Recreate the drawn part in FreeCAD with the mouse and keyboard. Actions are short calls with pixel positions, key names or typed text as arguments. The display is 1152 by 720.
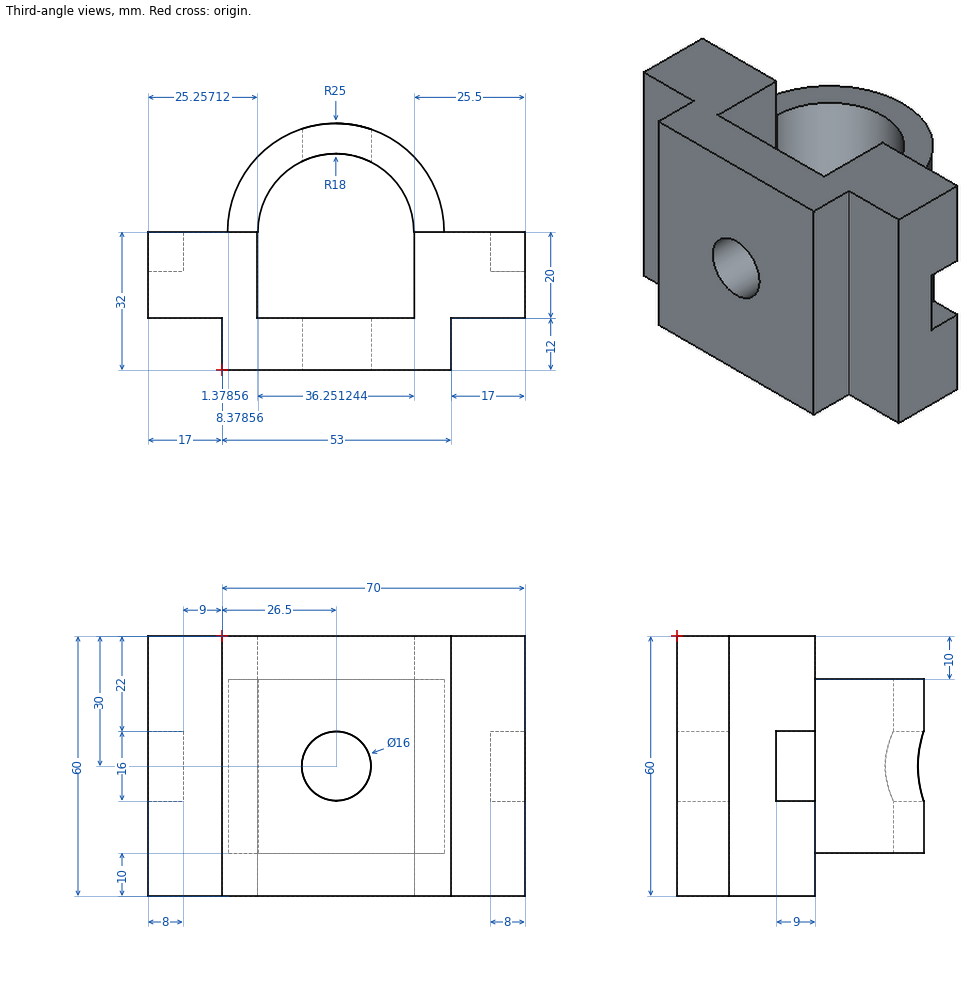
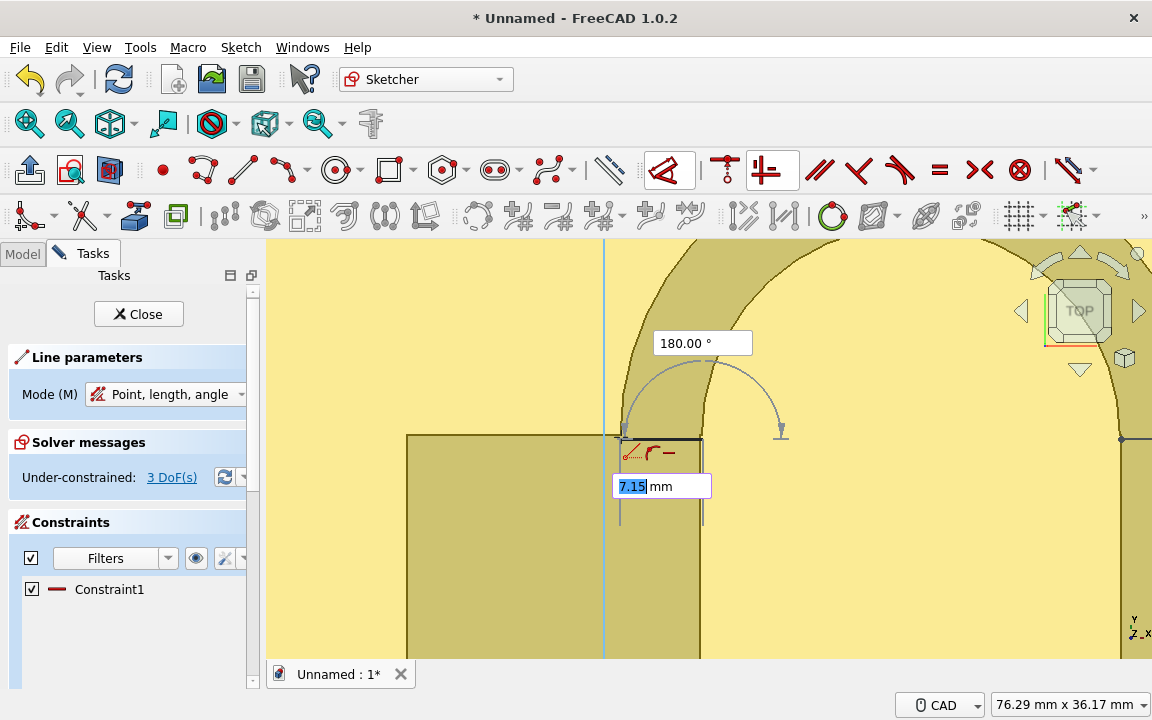
click(621, 436)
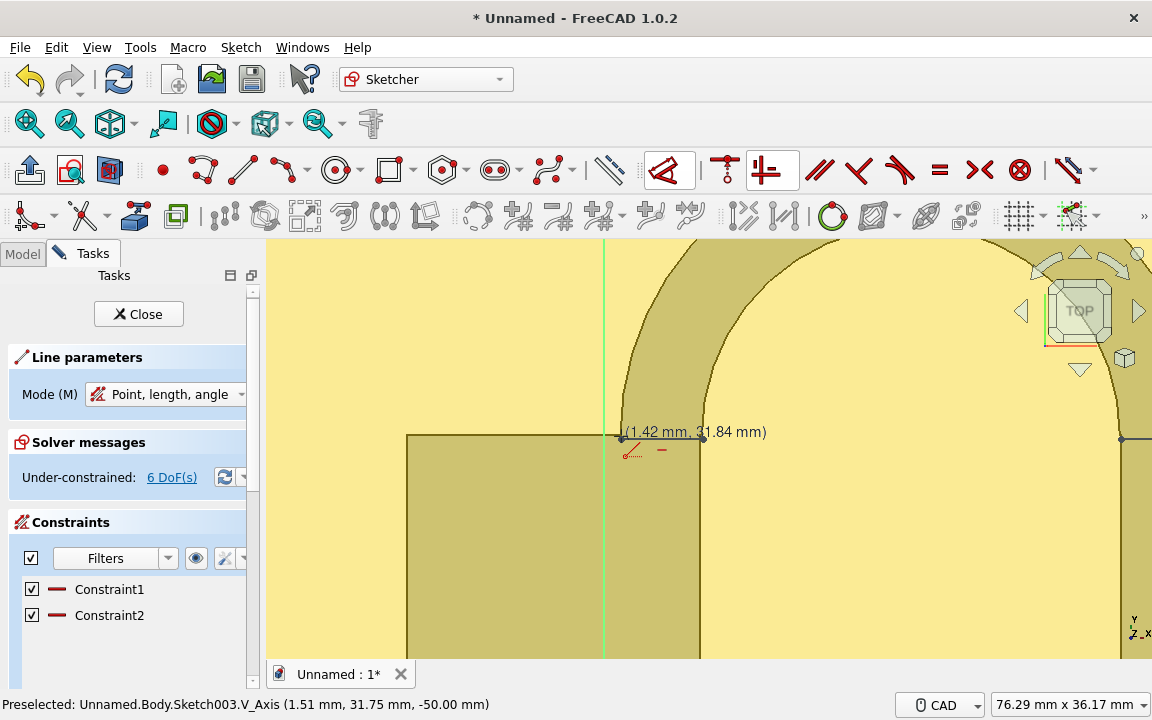
click(284, 170)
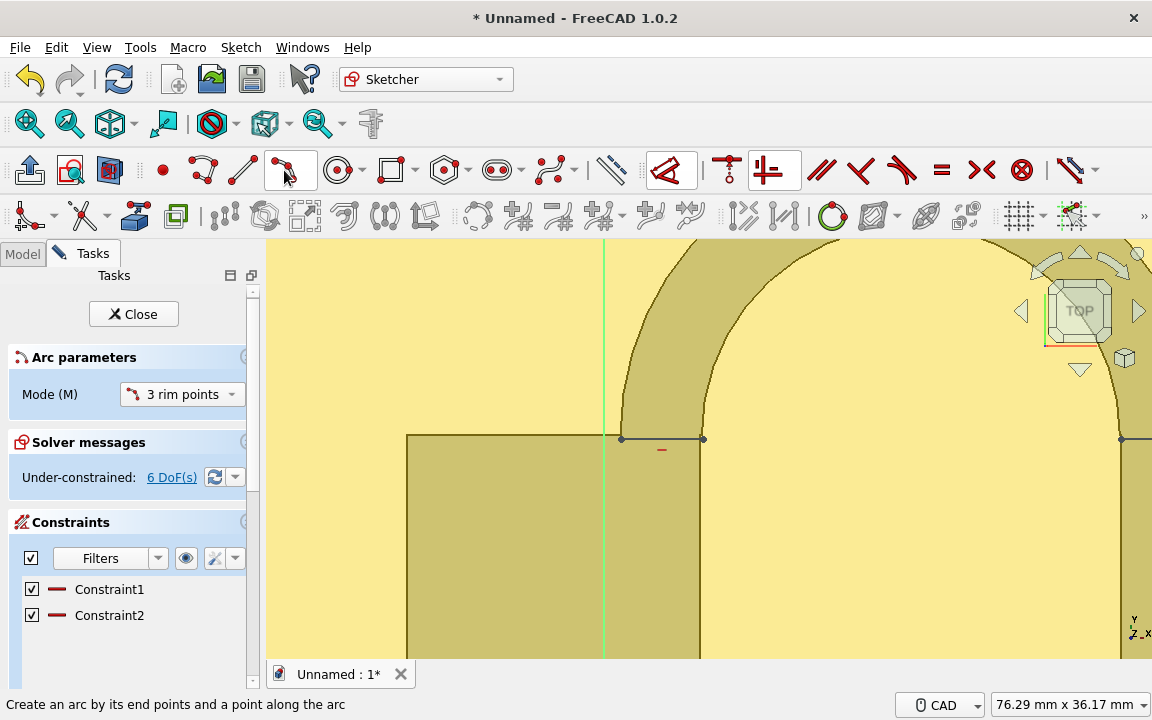
scroll(488, 433, down, 5)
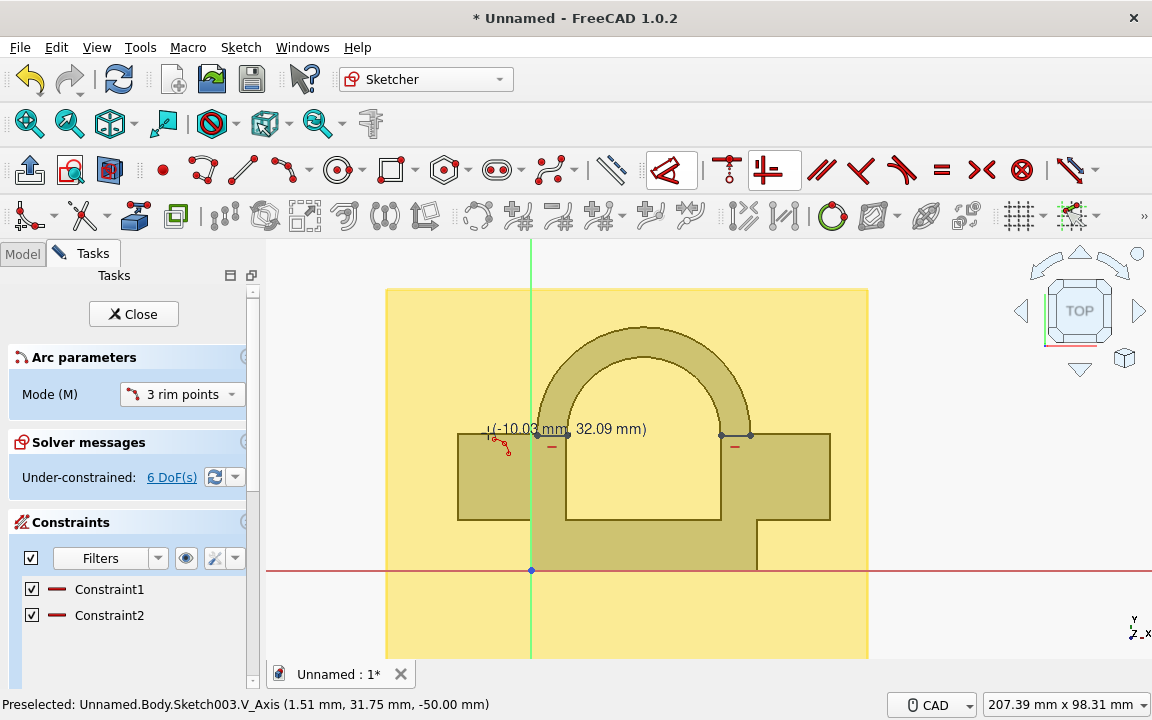
click(721, 436)
click(567, 436)
click(644, 357)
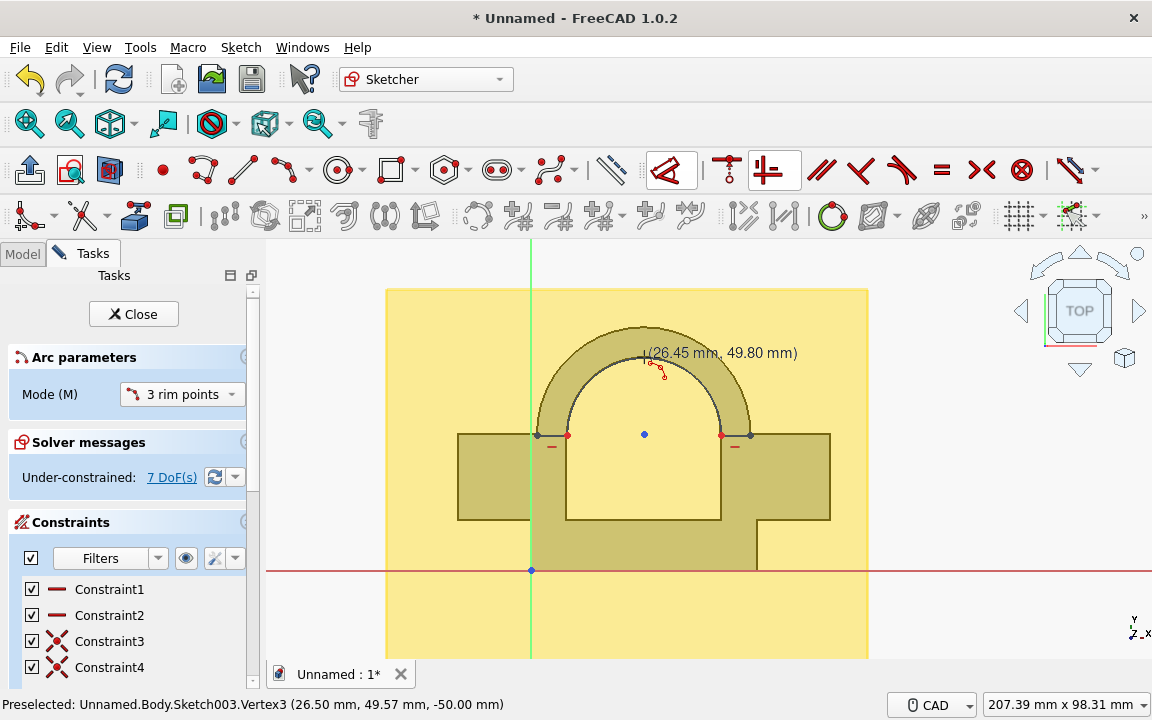
scroll(537, 434, up, 5)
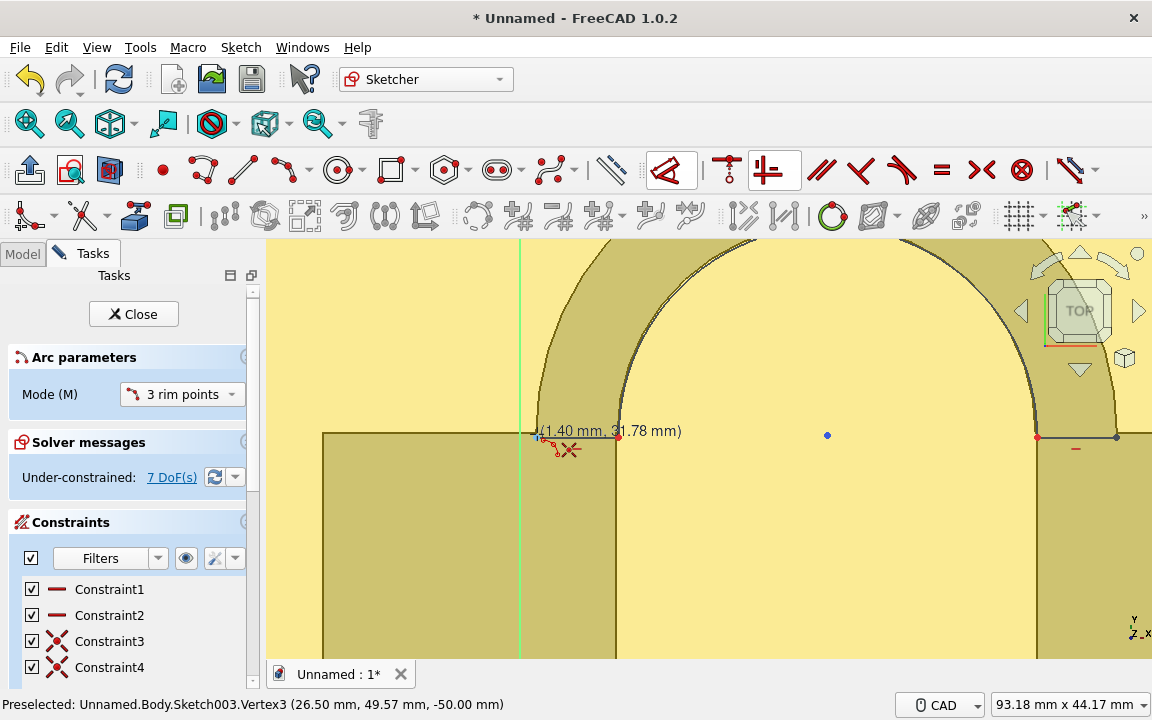
click(537, 438)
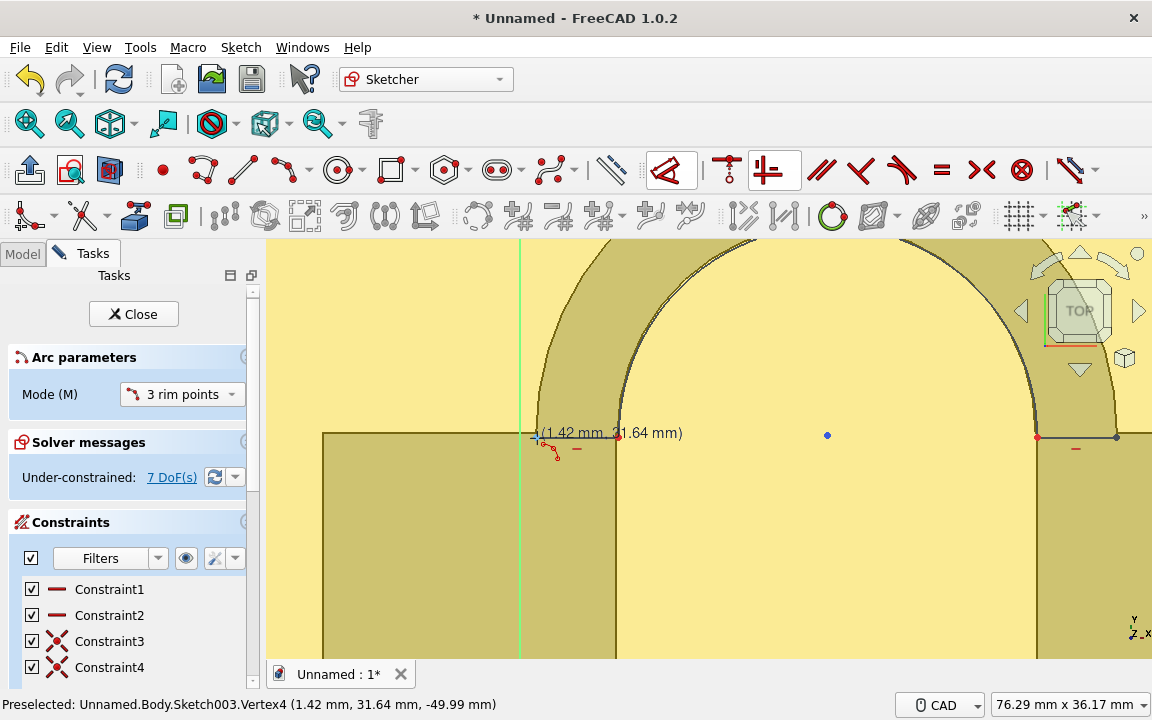
scroll(537, 434, down, 5)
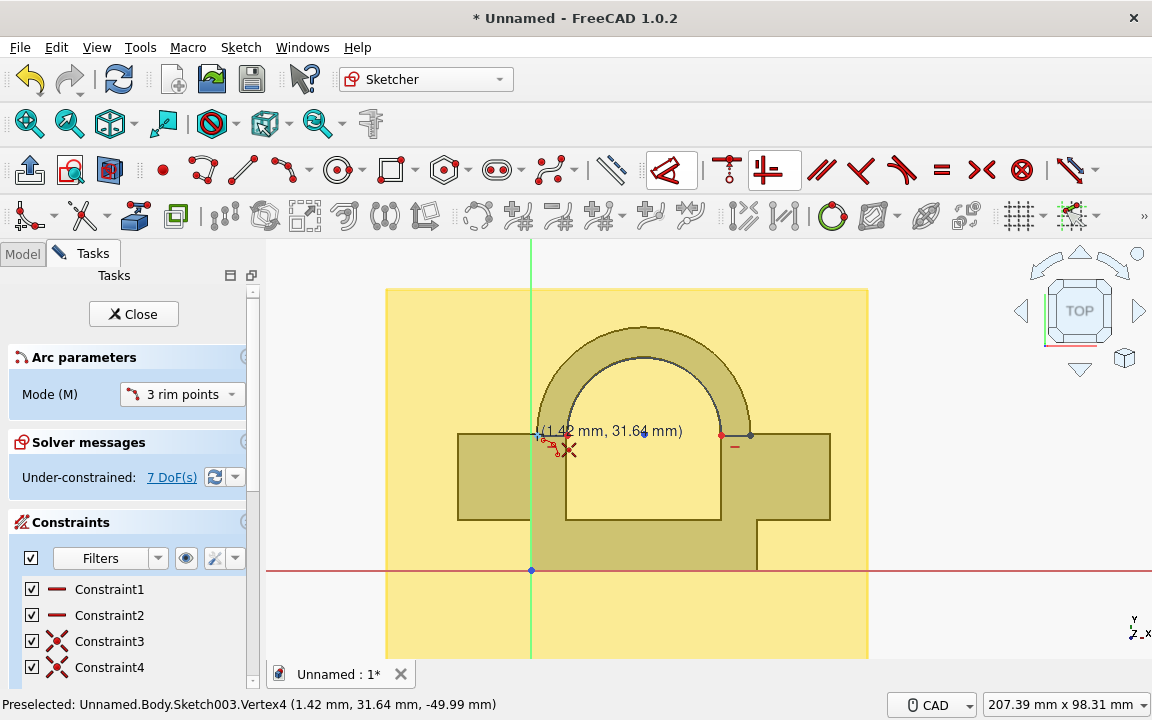
click(750, 436)
click(644, 327)
key(Escape)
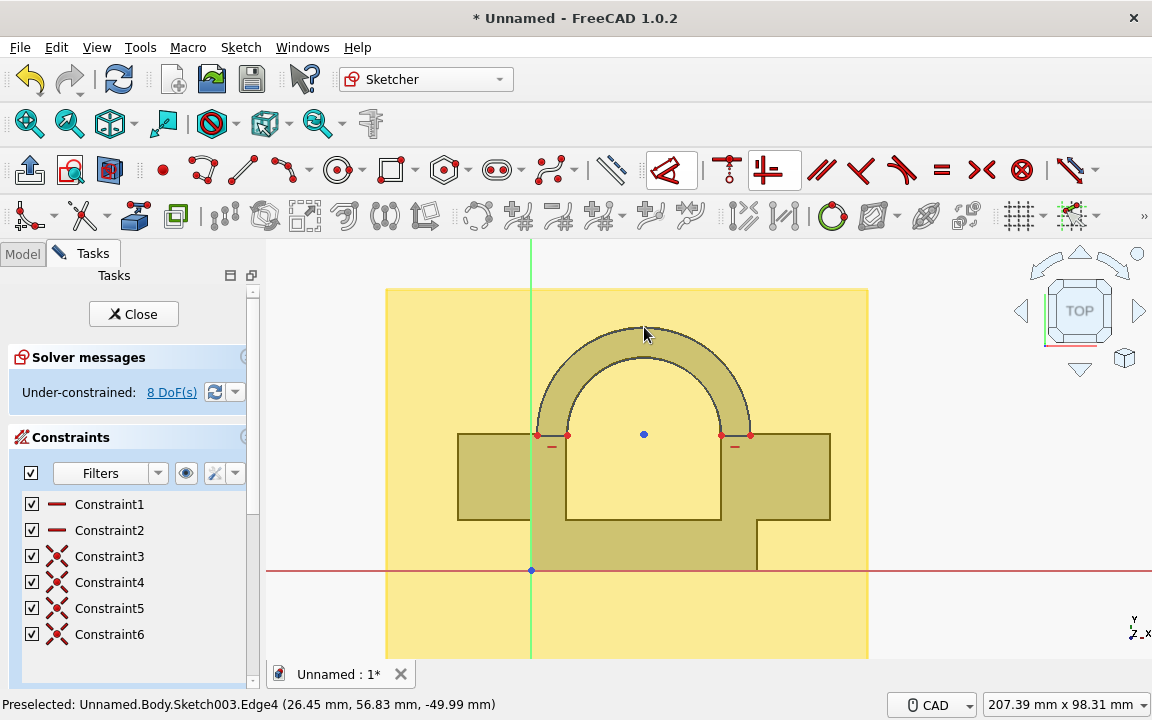
click(690, 373)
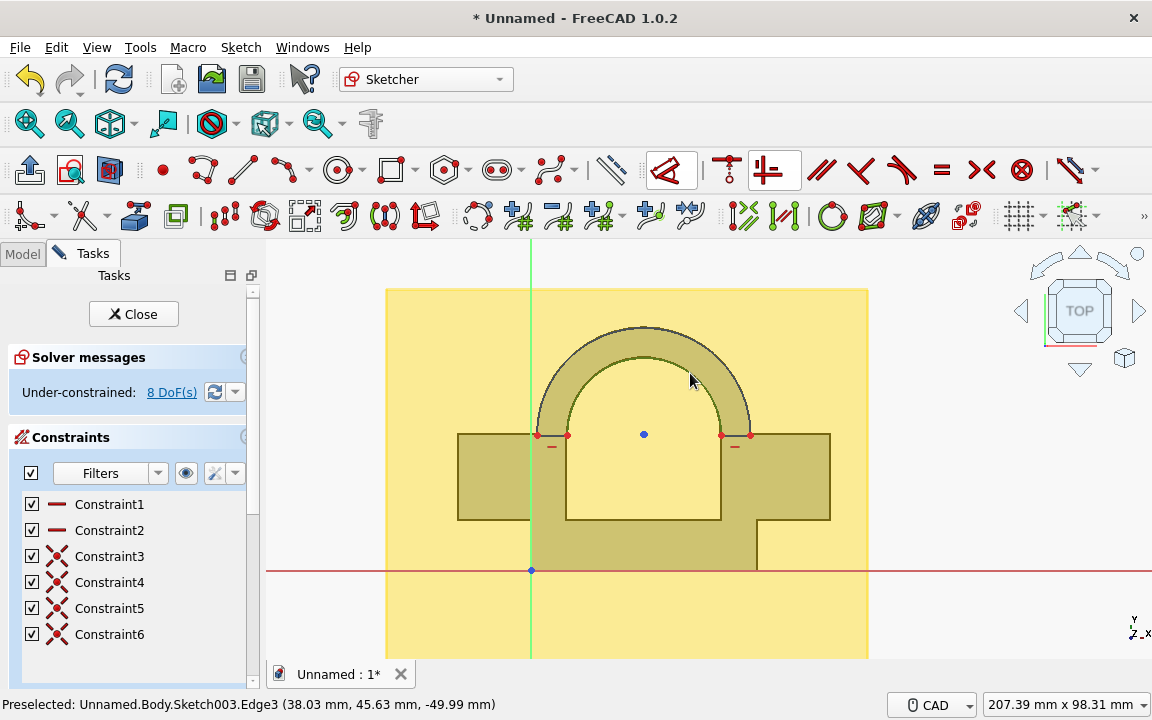
click(707, 349)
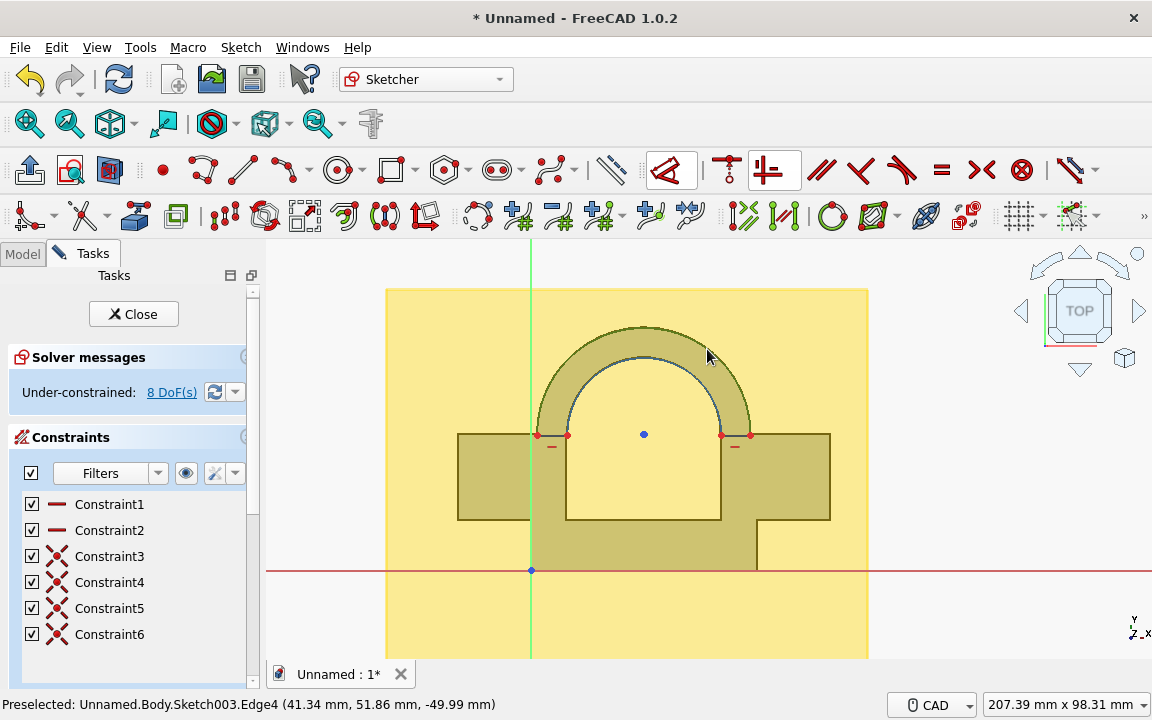
key(c)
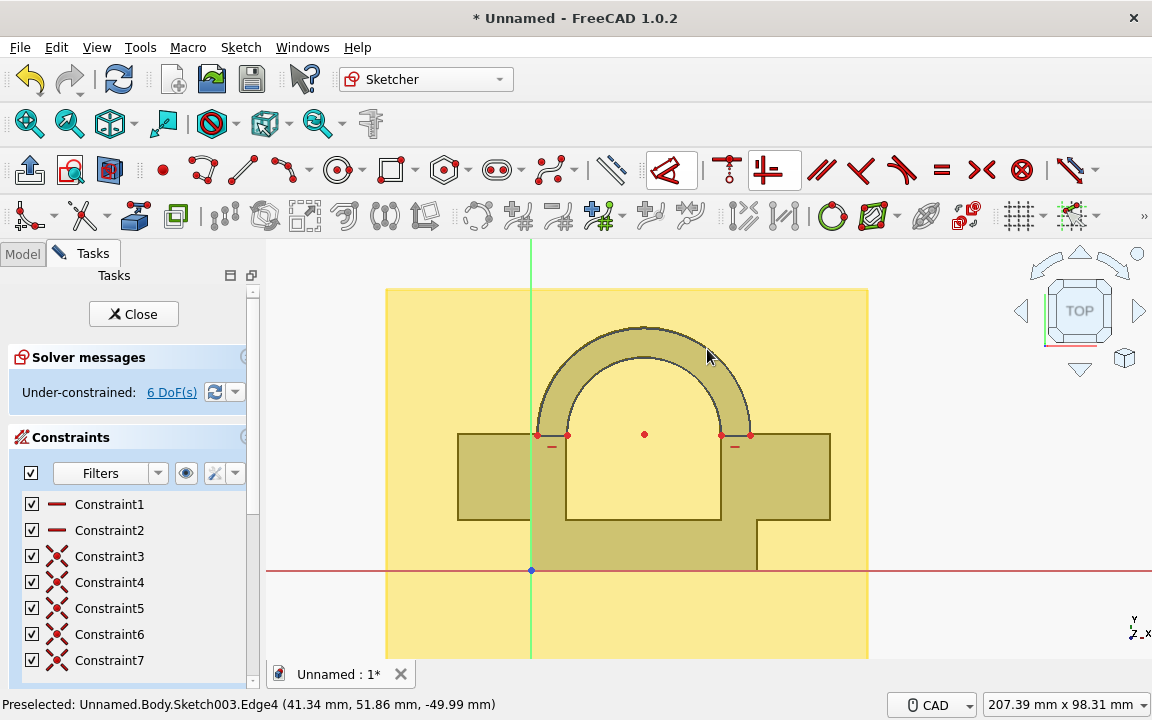
click(690, 373)